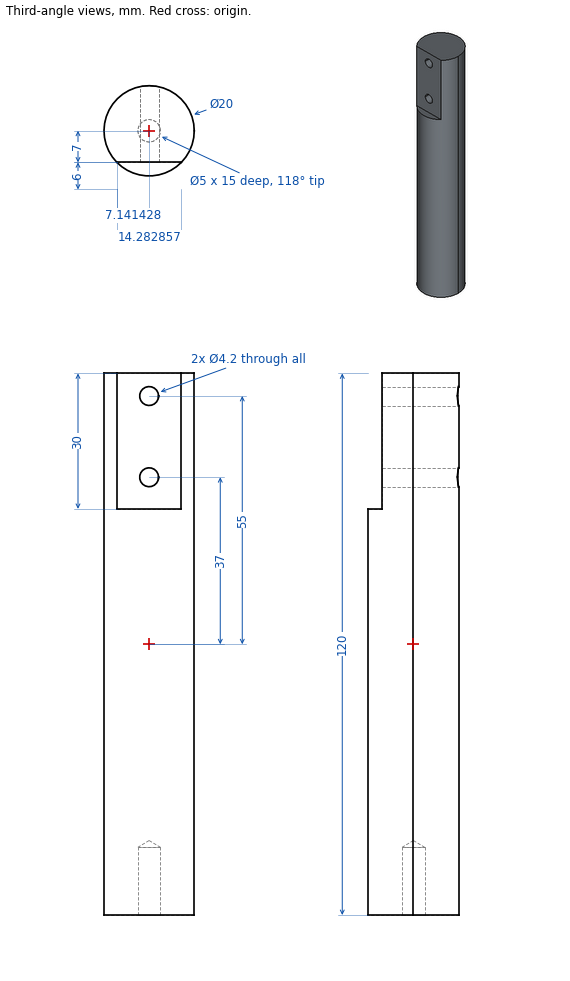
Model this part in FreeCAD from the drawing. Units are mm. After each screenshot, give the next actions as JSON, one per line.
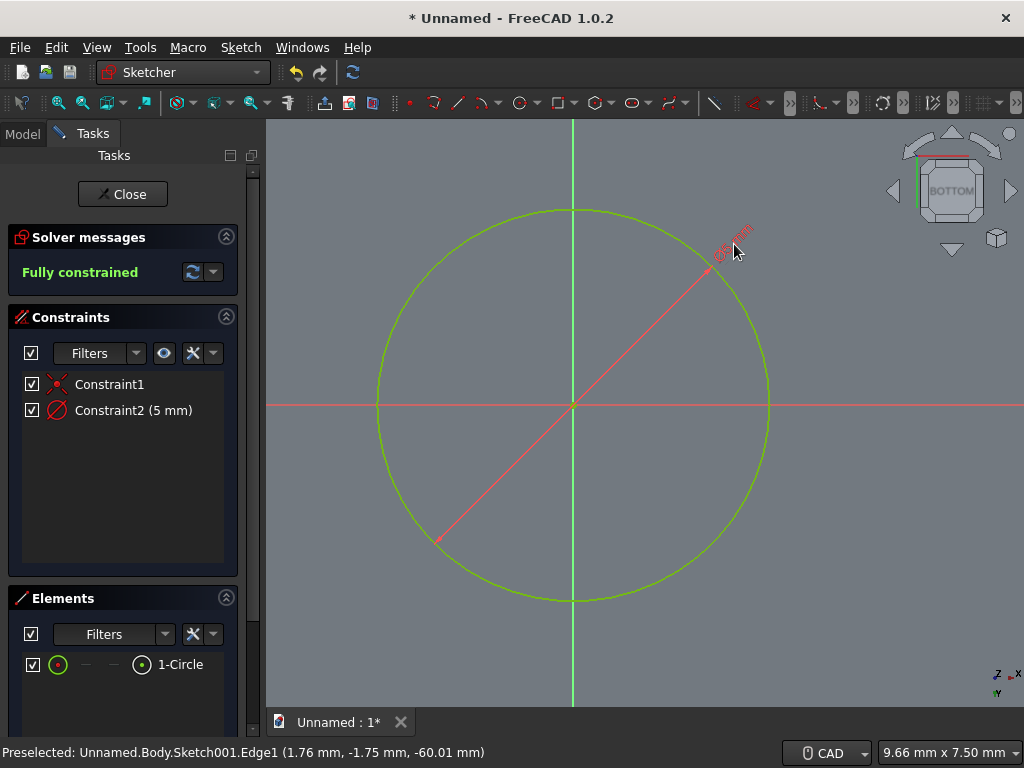
{"action": "left_click", "coordinate": [123, 194]}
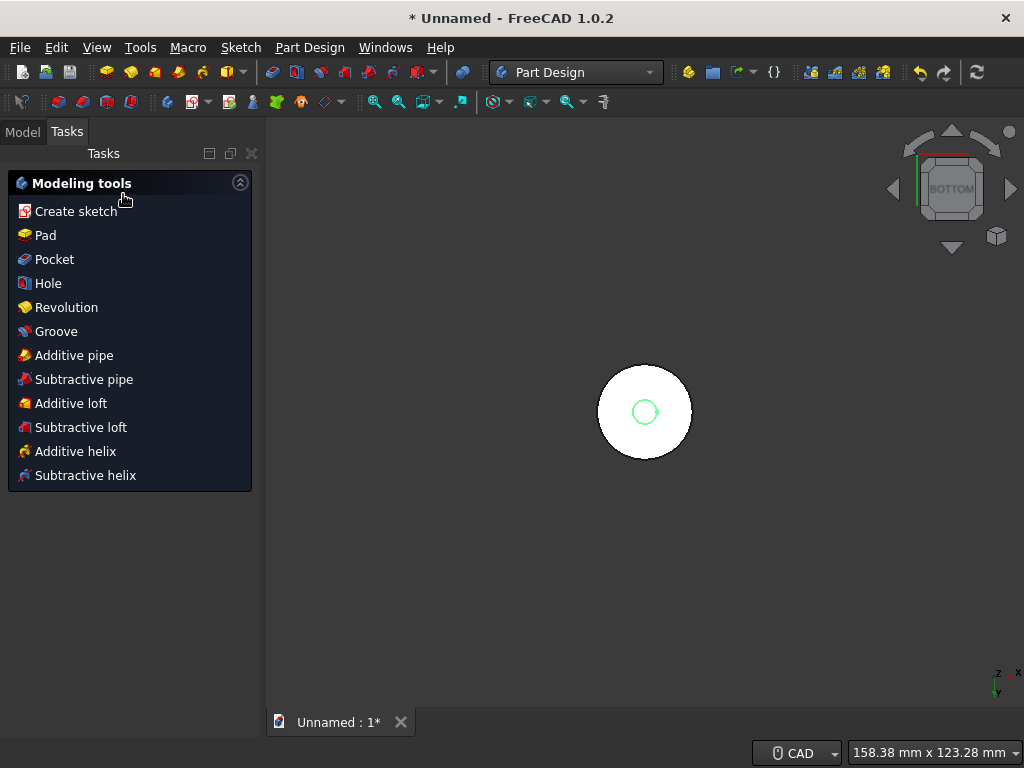
{"action": "left_click", "coordinate": [298, 72]}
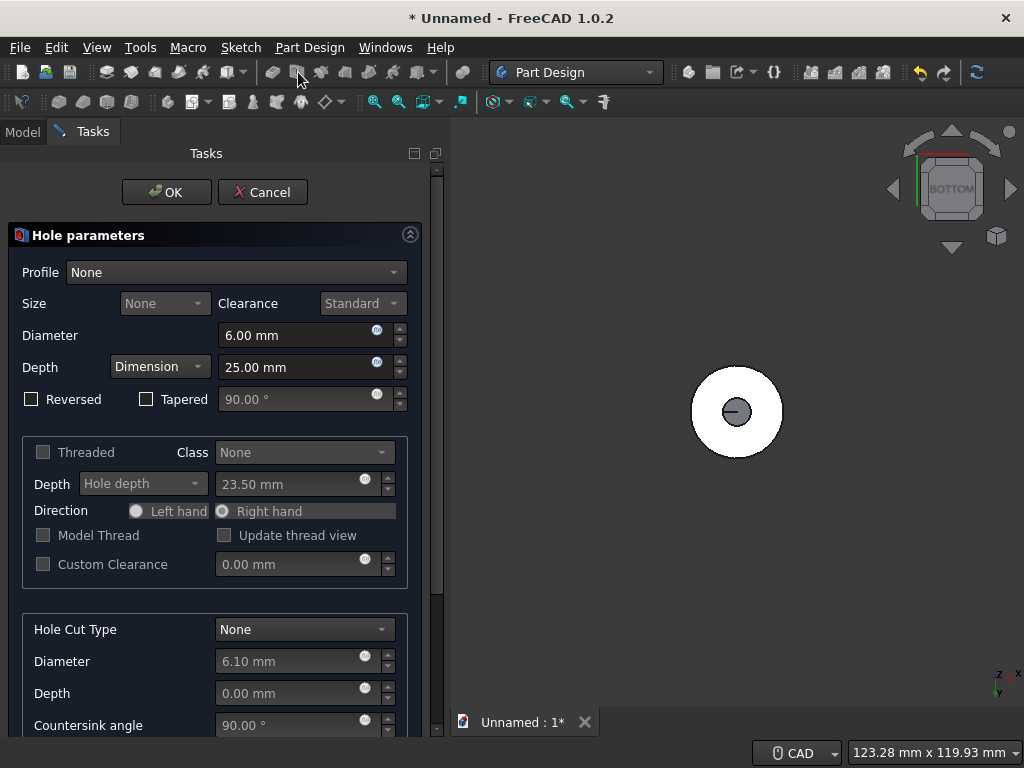
{"action": "triple_click", "coordinate": [305, 335]}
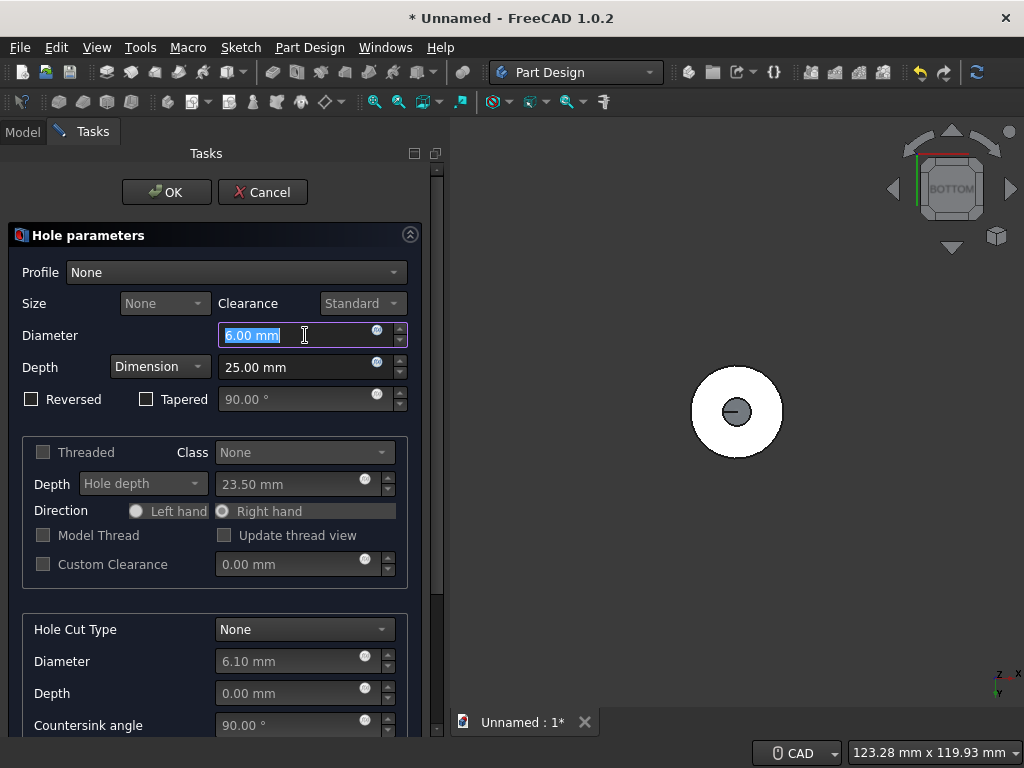
{"action": "type", "text": "5"}
{"action": "key", "text": "Tab"}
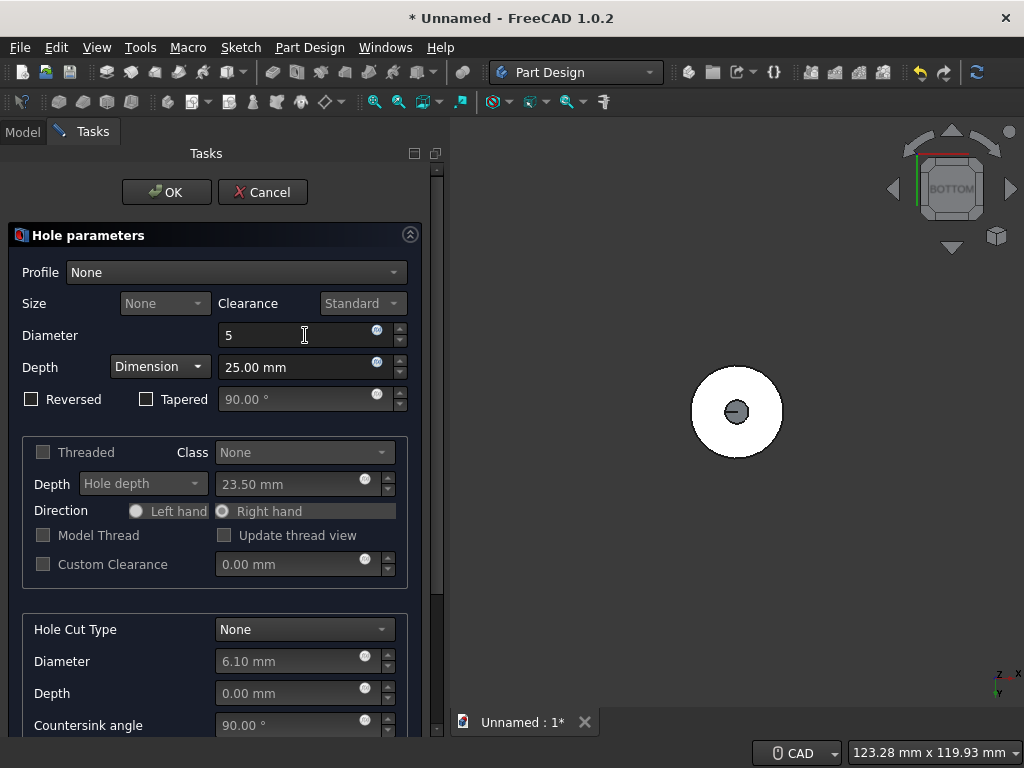
{"action": "triple_click", "coordinate": [305, 367]}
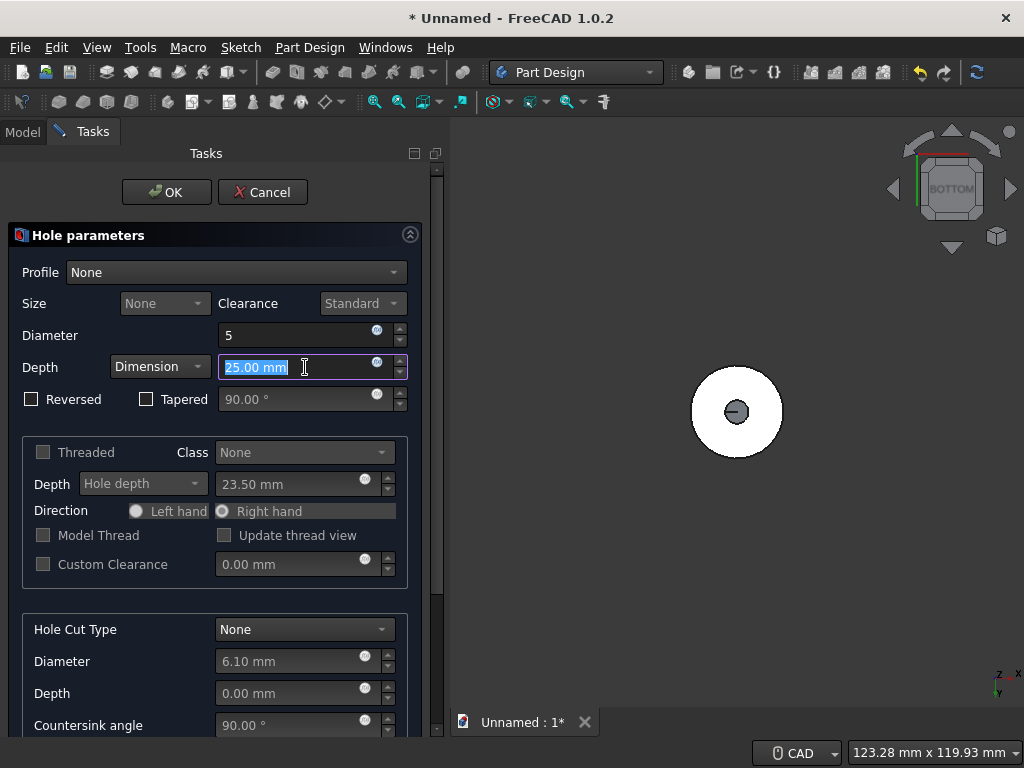
{"action": "type", "text": "15"}
{"action": "key", "text": "Tab"}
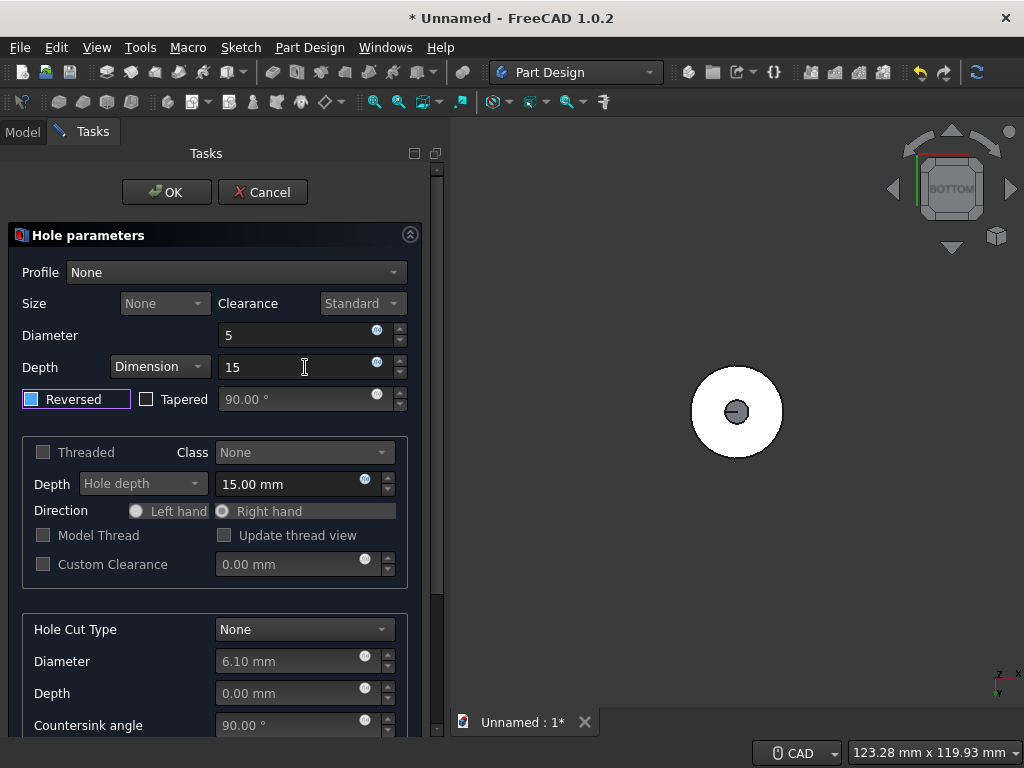
{"action": "left_click", "coordinate": [167, 192]}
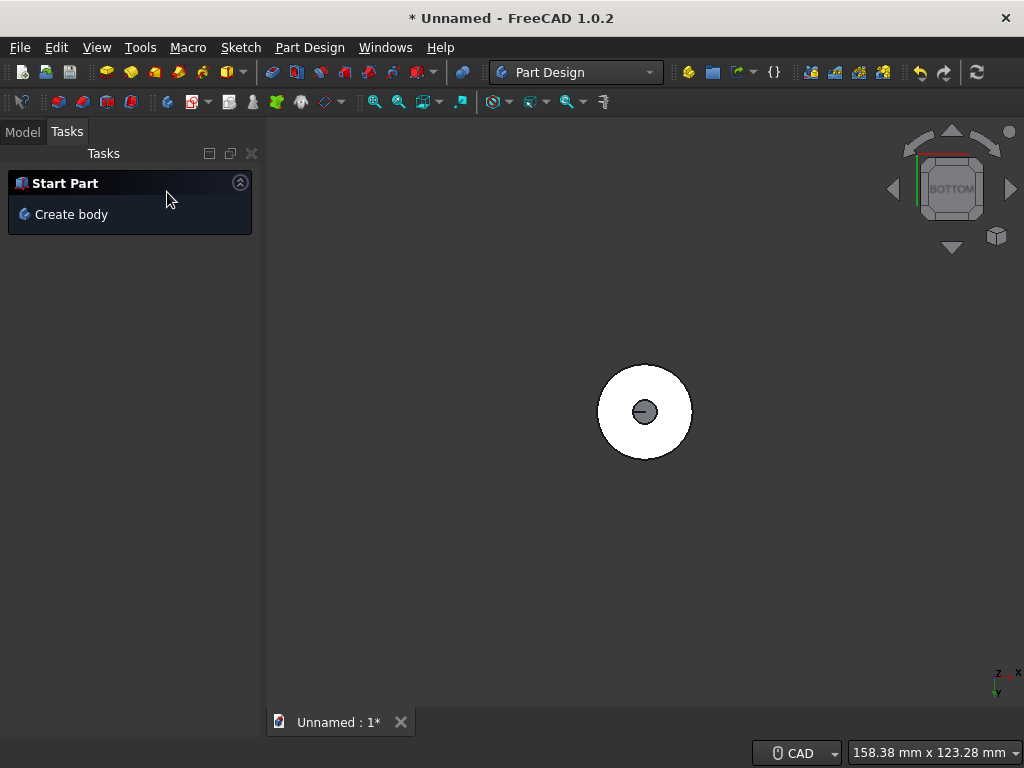
{"action": "left_click", "coordinate": [376, 102]}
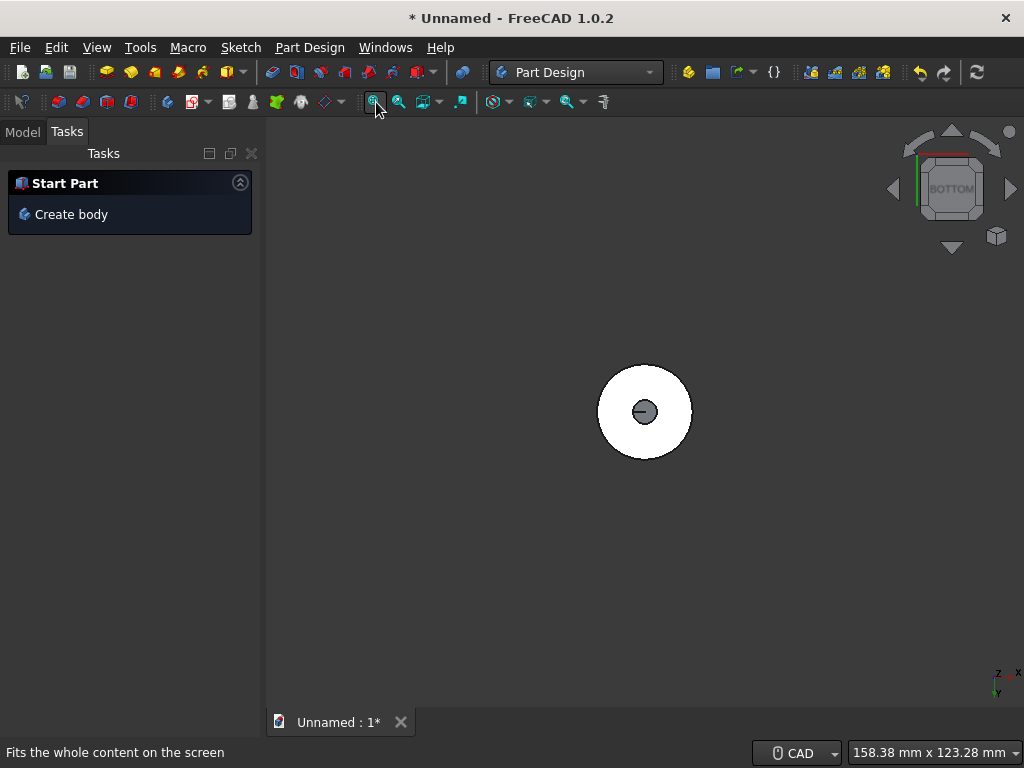
{"action": "key", "text": "0"}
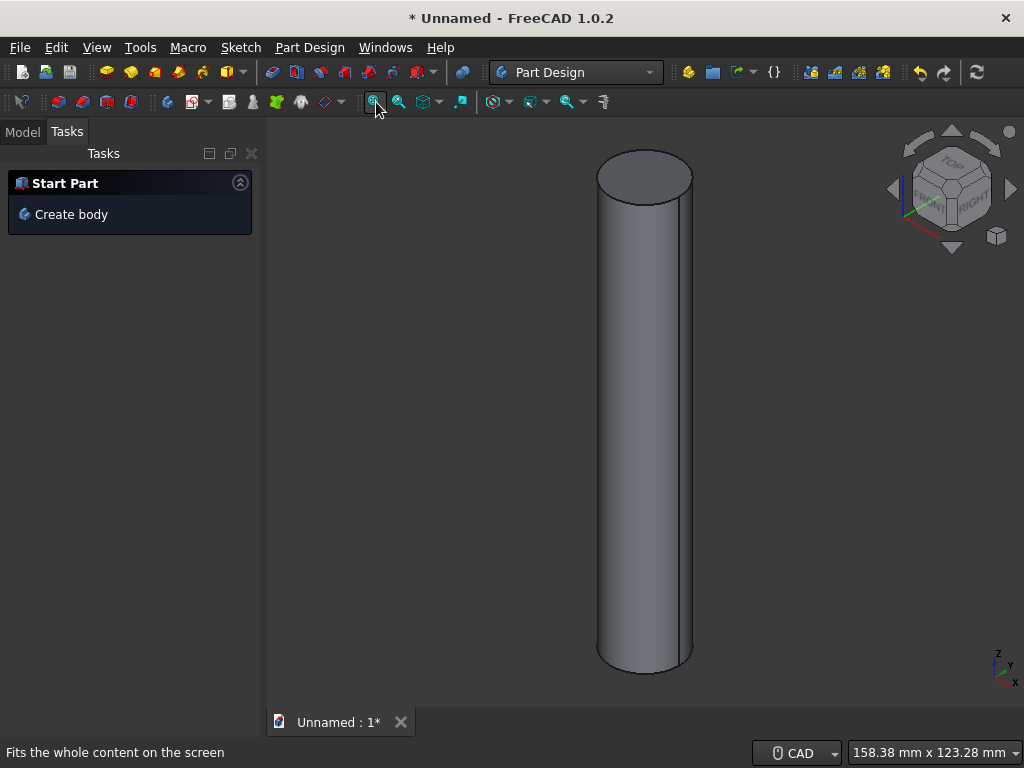
{"action": "left_click", "coordinate": [645, 176]}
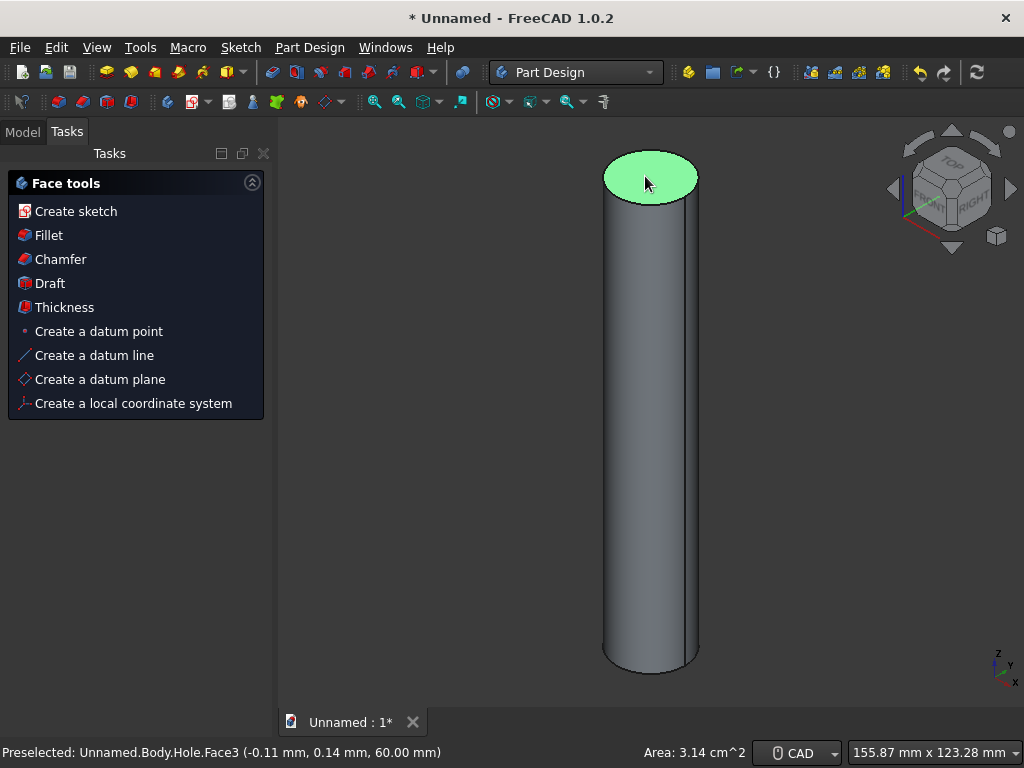
{"action": "left_click", "coordinate": [192, 102]}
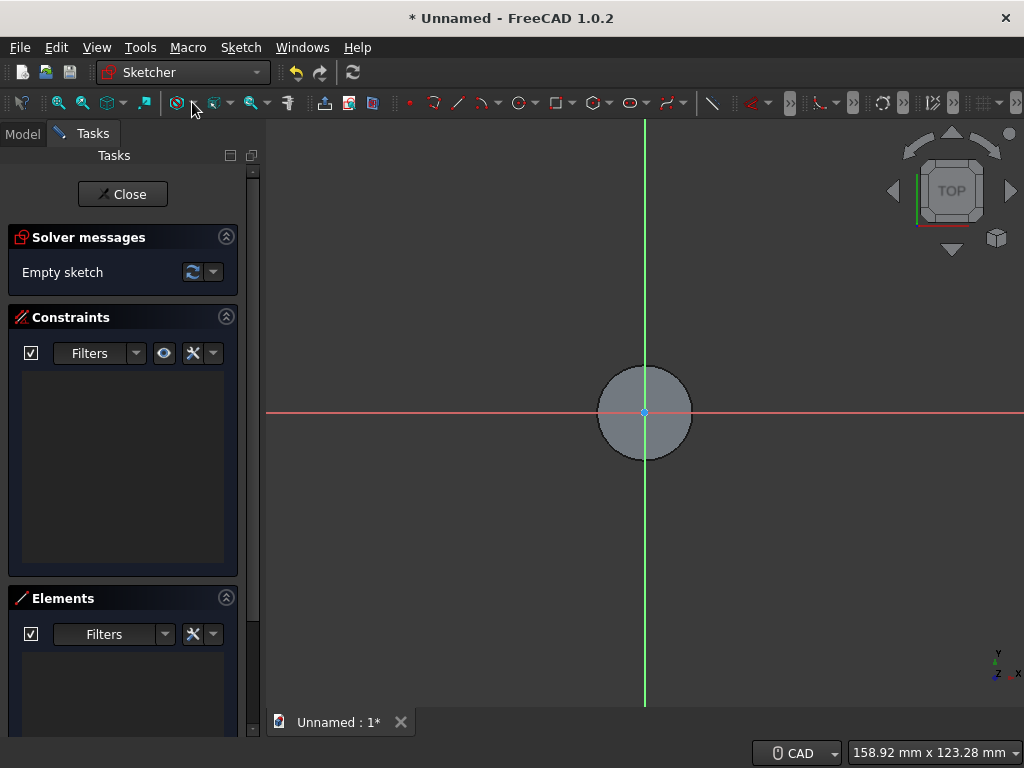
{"action": "scroll", "coordinate": [658, 450], "scroll_direction": "up", "scroll_amount": 9}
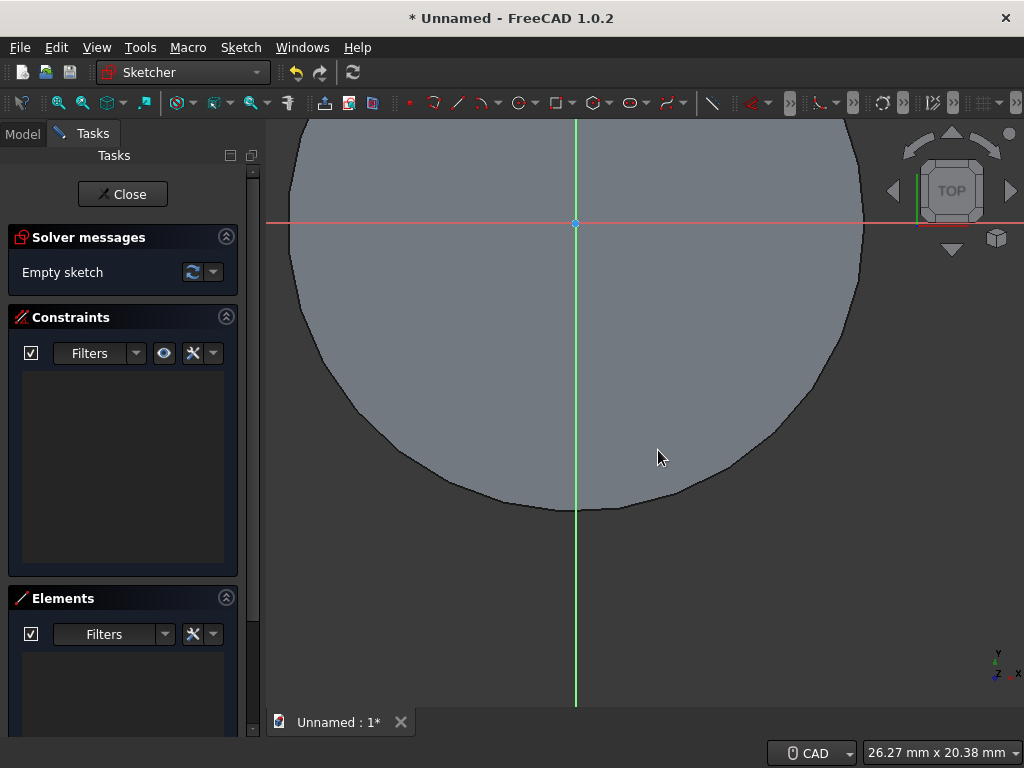
{"action": "left_click", "coordinate": [556, 104]}